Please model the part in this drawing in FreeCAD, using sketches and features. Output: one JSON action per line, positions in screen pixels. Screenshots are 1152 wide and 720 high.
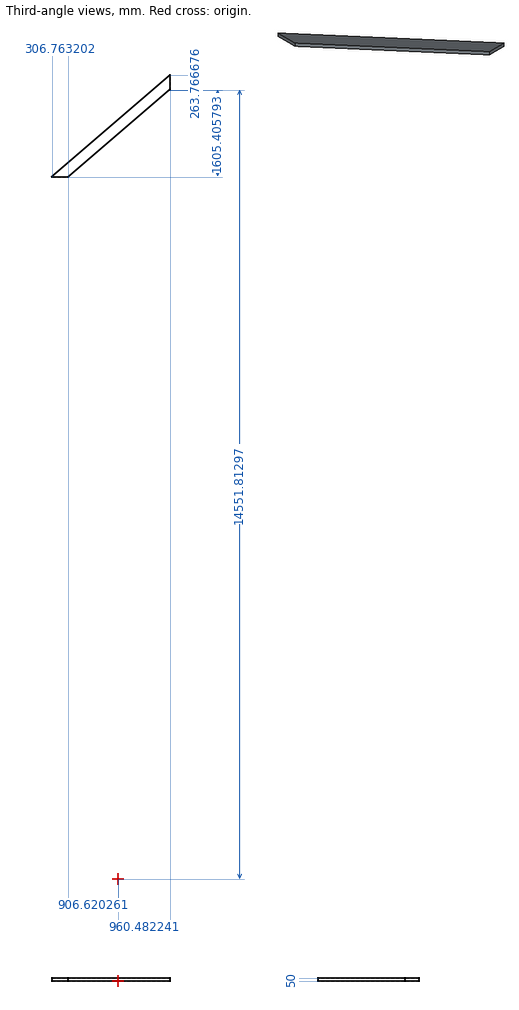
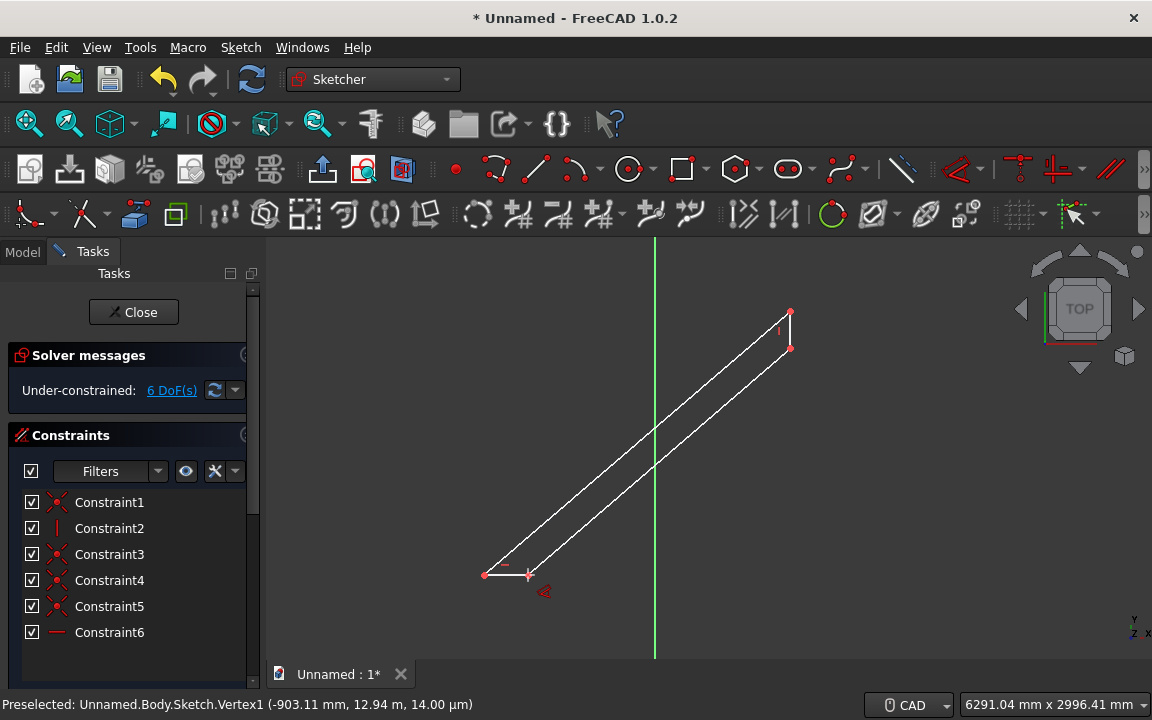
{"action": "scroll", "coordinate": [790, 338], "scroll_direction": "up", "scroll_amount": 2}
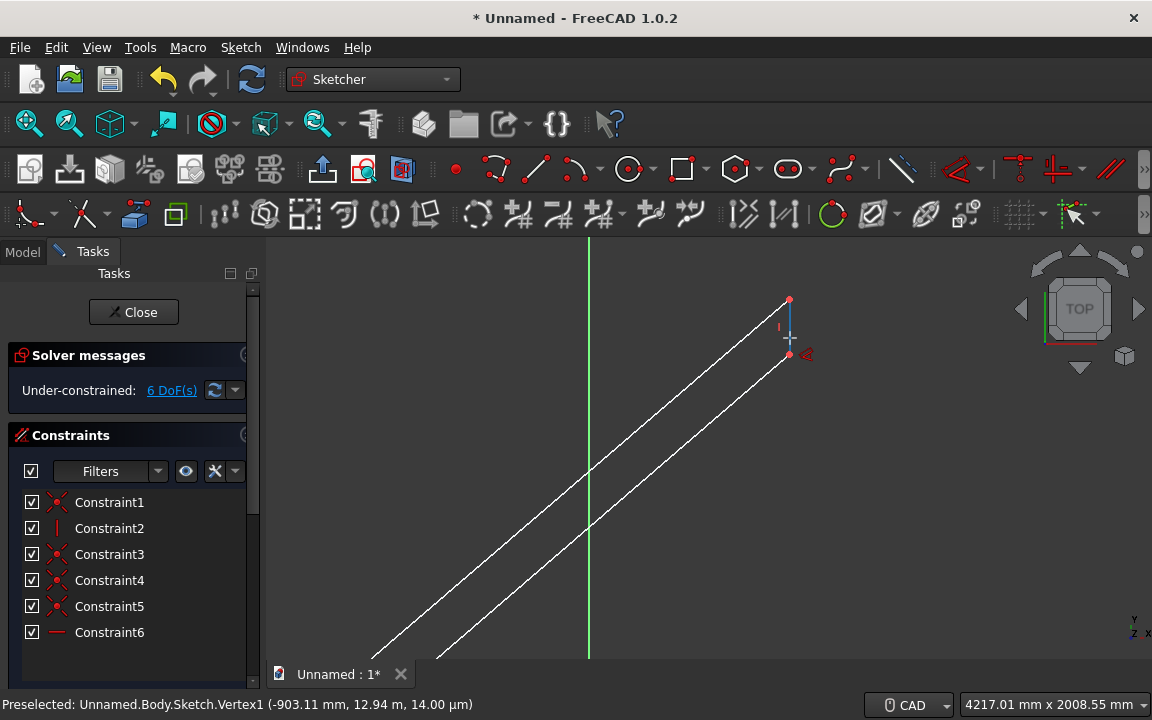
{"action": "left_click", "coordinate": [790, 338]}
{"action": "left_click", "coordinate": [824, 327]}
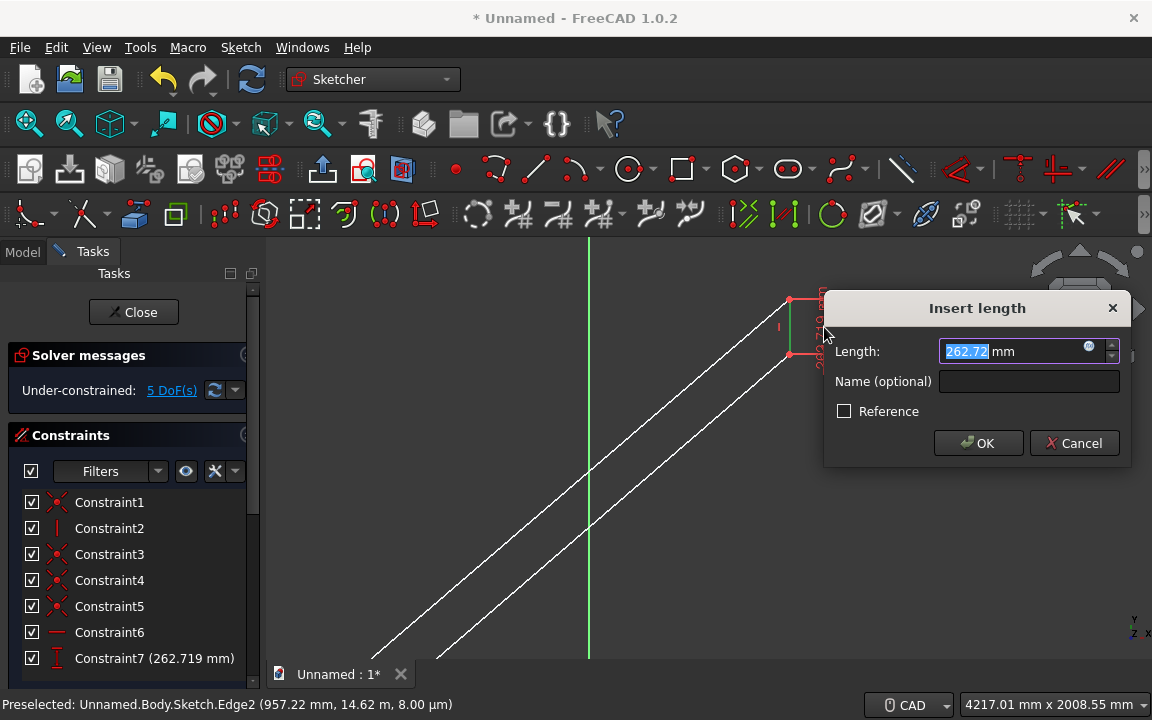
{"action": "type", "text": "263.766676"}
{"action": "key", "text": "Return"}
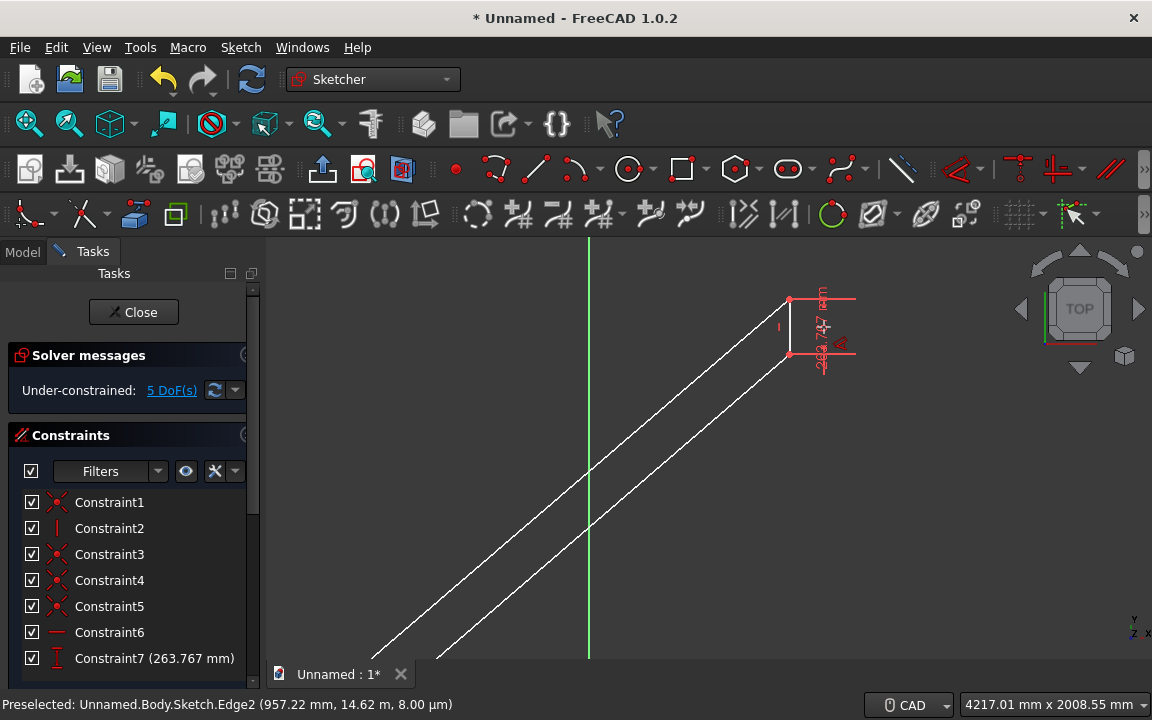
{"action": "scroll", "coordinate": [800, 355], "scroll_direction": "down", "scroll_amount": 2}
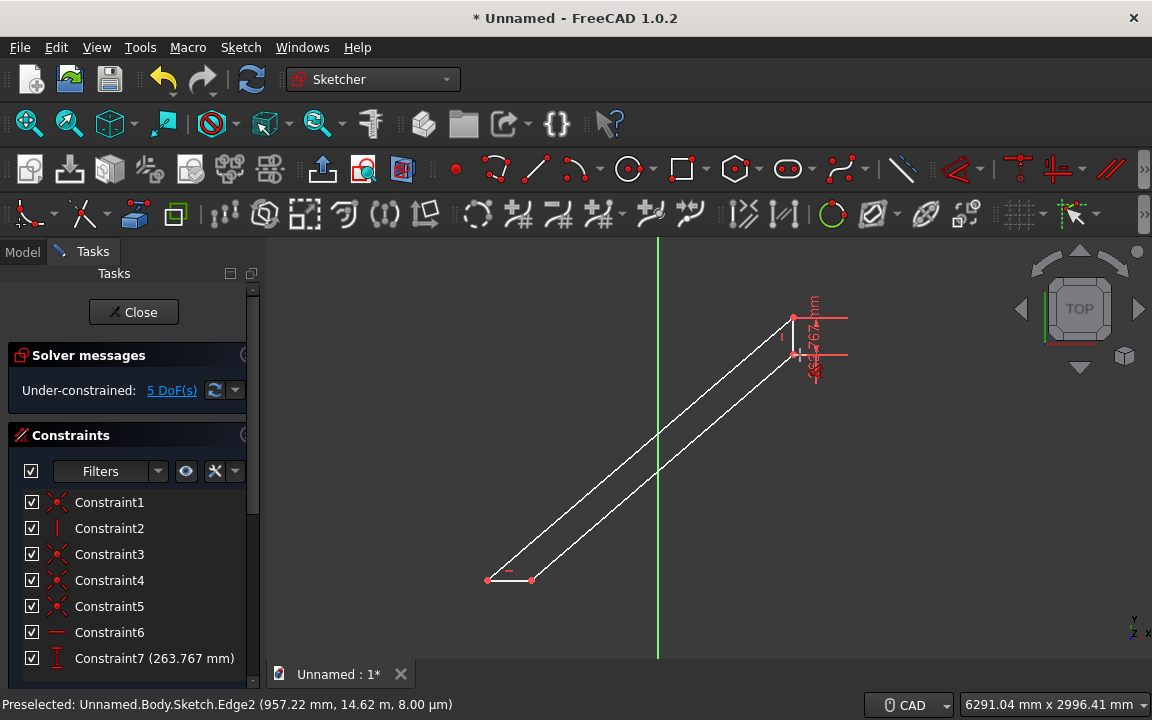
{"action": "scroll", "coordinate": [501, 581], "scroll_direction": "up", "scroll_amount": 3}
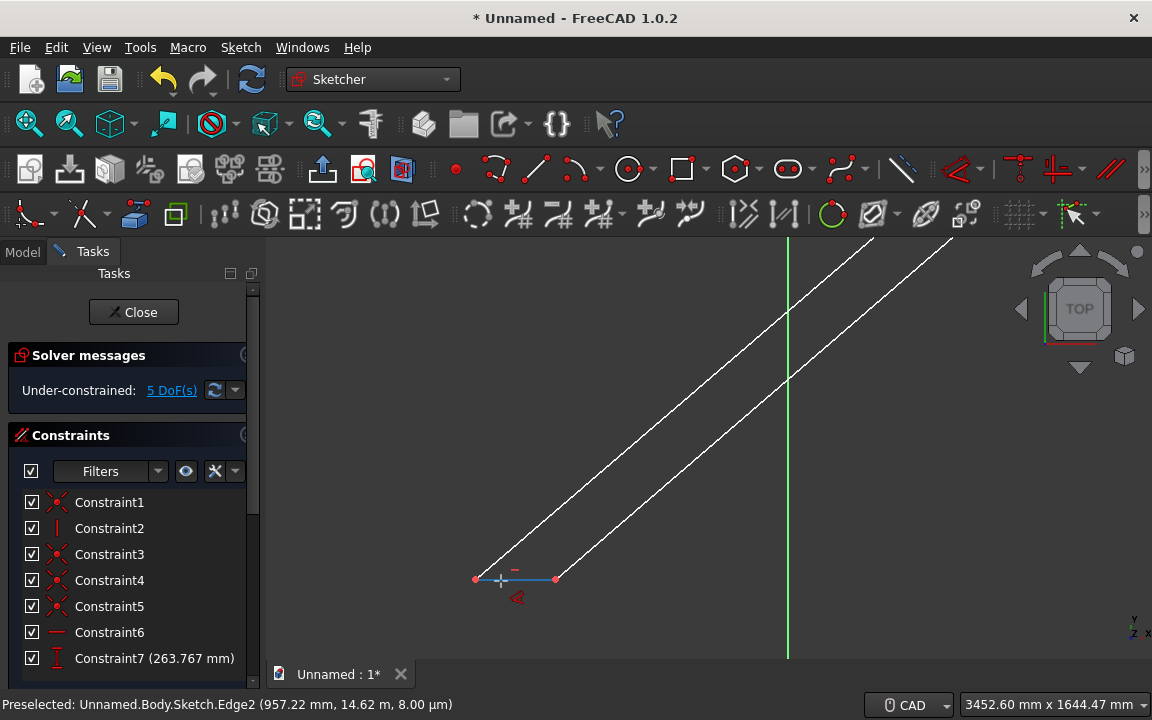
{"action": "left_click", "coordinate": [500, 580]}
{"action": "left_click", "coordinate": [516, 614]}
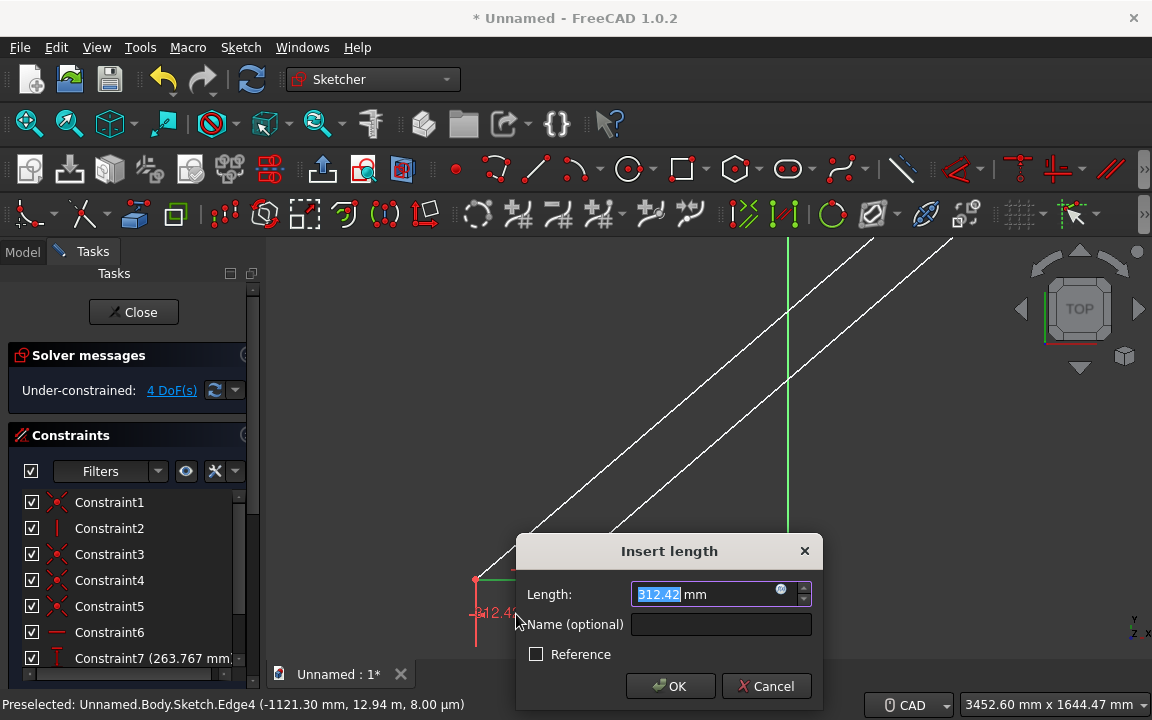
{"action": "type", "text": "306.763202"}
{"action": "key", "text": "Return"}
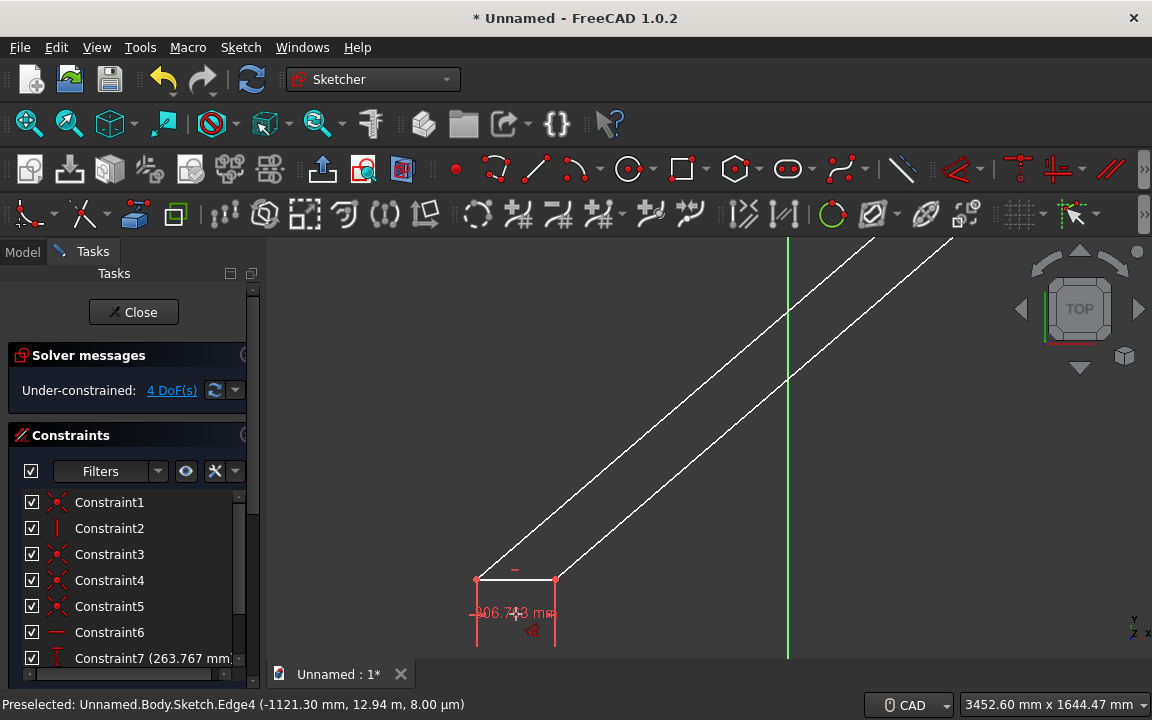
{"action": "left_click", "coordinate": [555, 580]}
{"action": "left_click", "coordinate": [672, 546]}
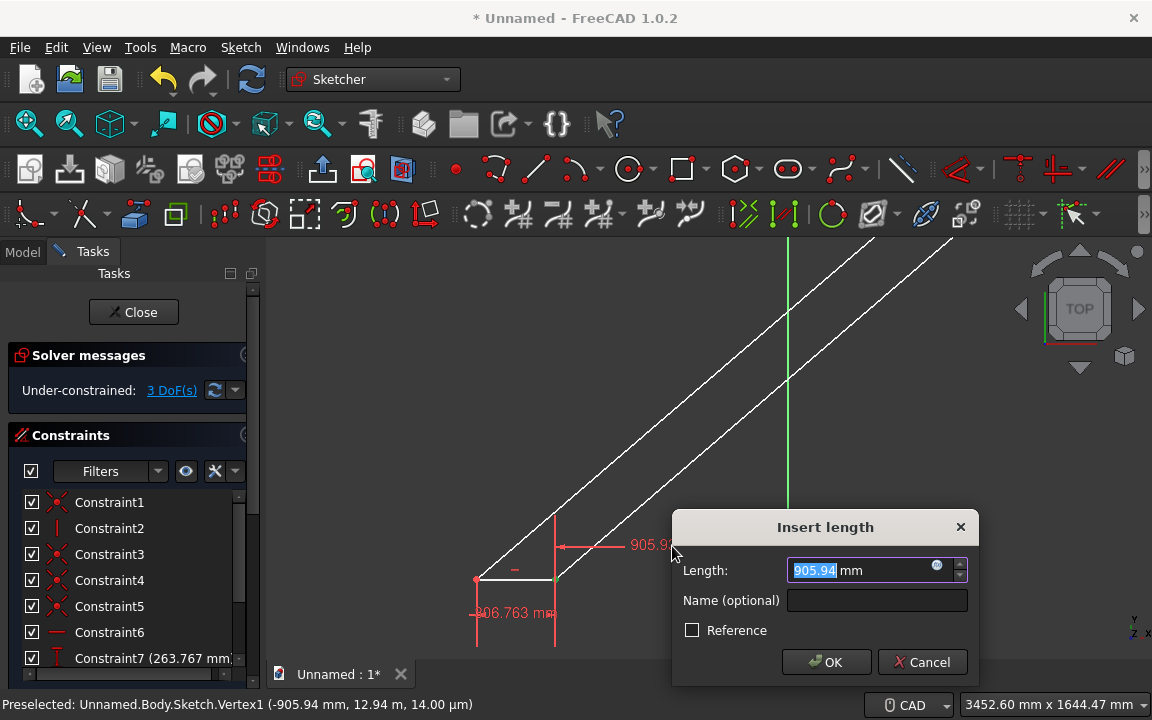
{"action": "type", "text": "906.620261"}
{"action": "key", "text": "Return"}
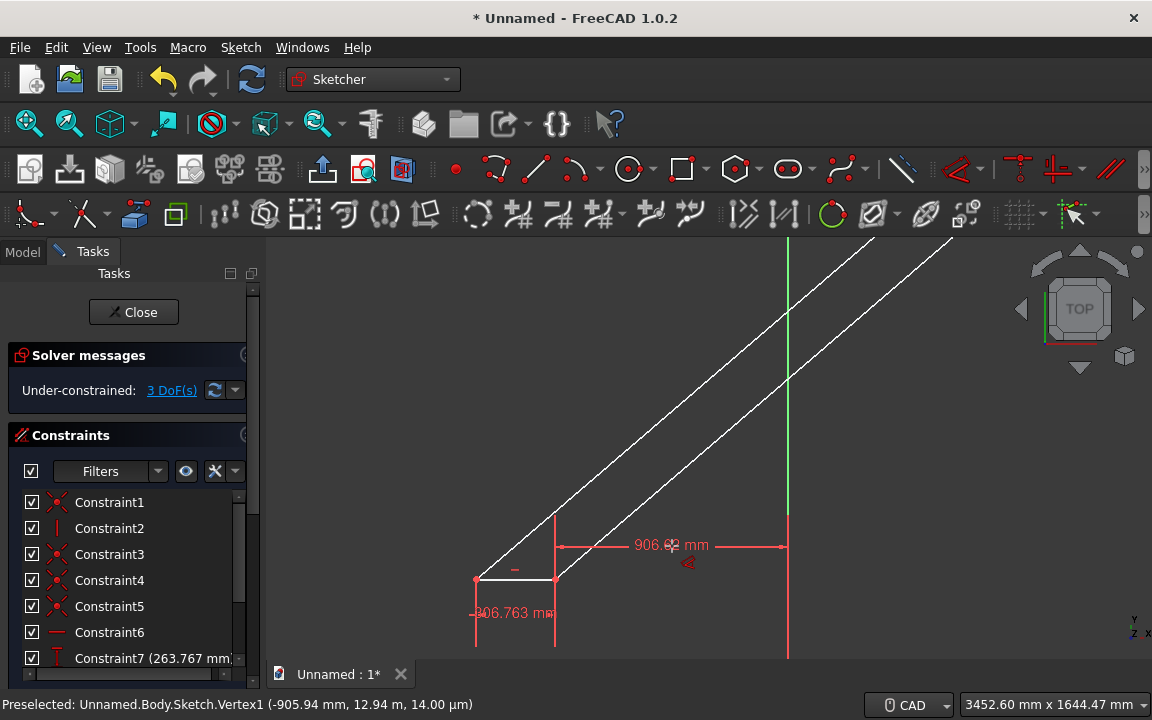
{"action": "scroll", "coordinate": [501, 582], "scroll_direction": "down", "scroll_amount": 3}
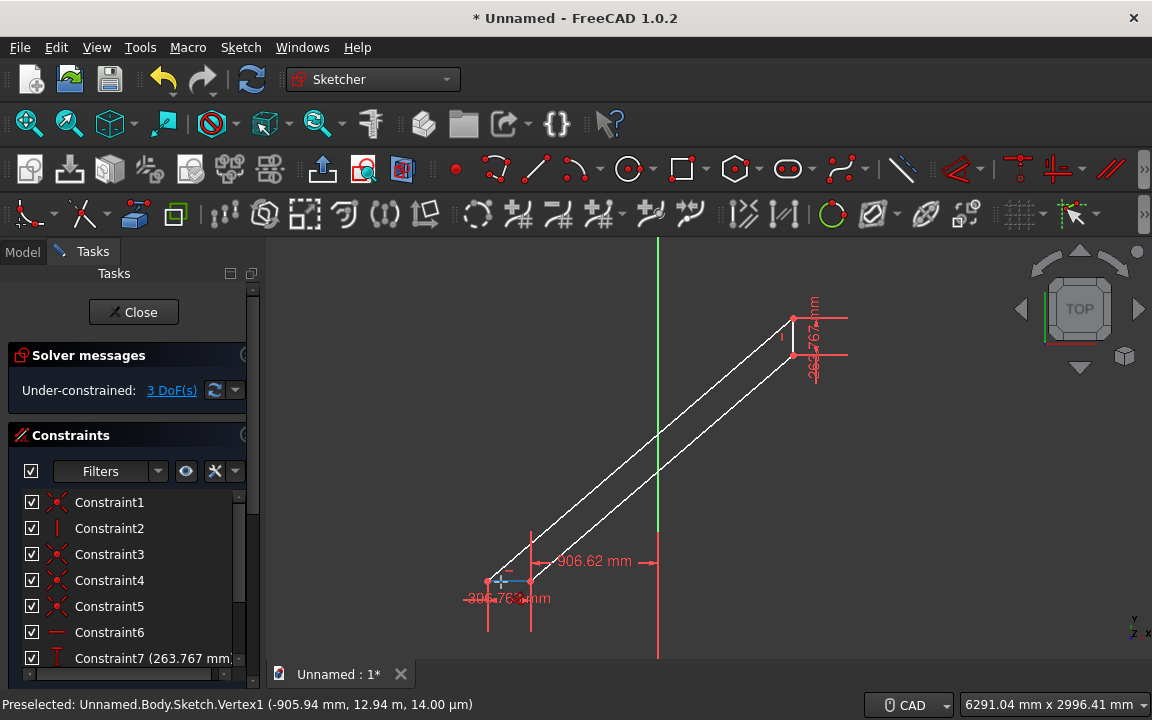
{"action": "left_click", "coordinate": [793, 355]}
{"action": "left_click", "coordinate": [726, 321]}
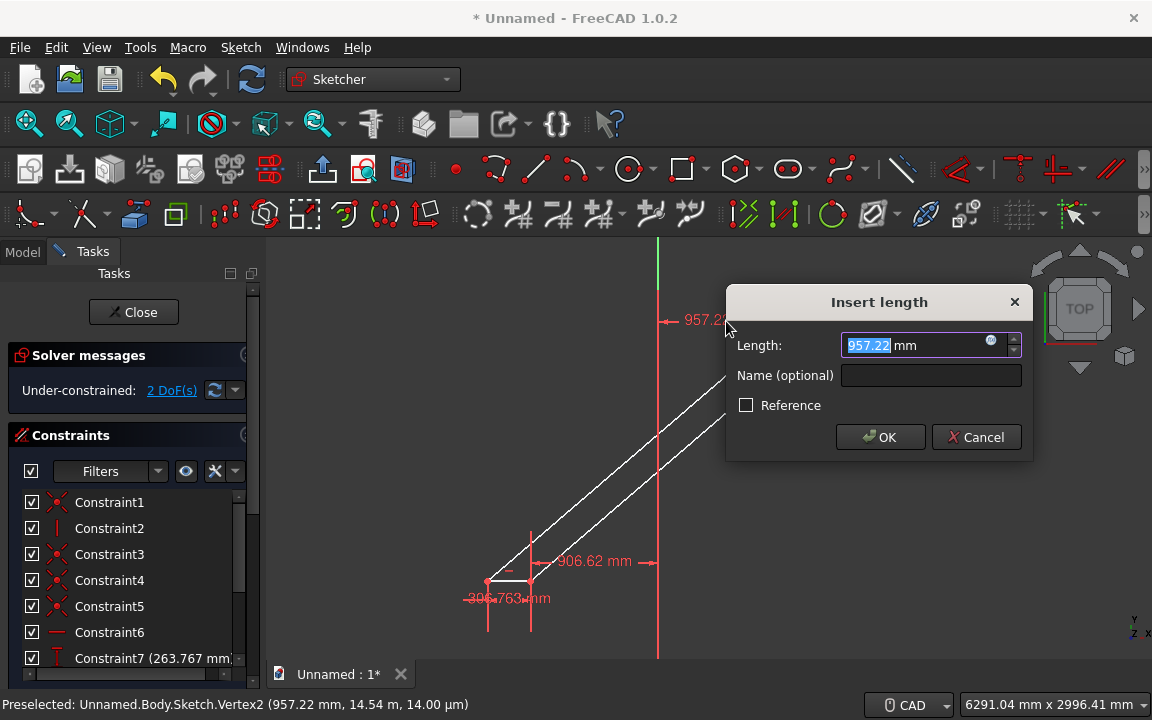
{"action": "type", "text": "960.482241"}
{"action": "key", "text": "Return"}